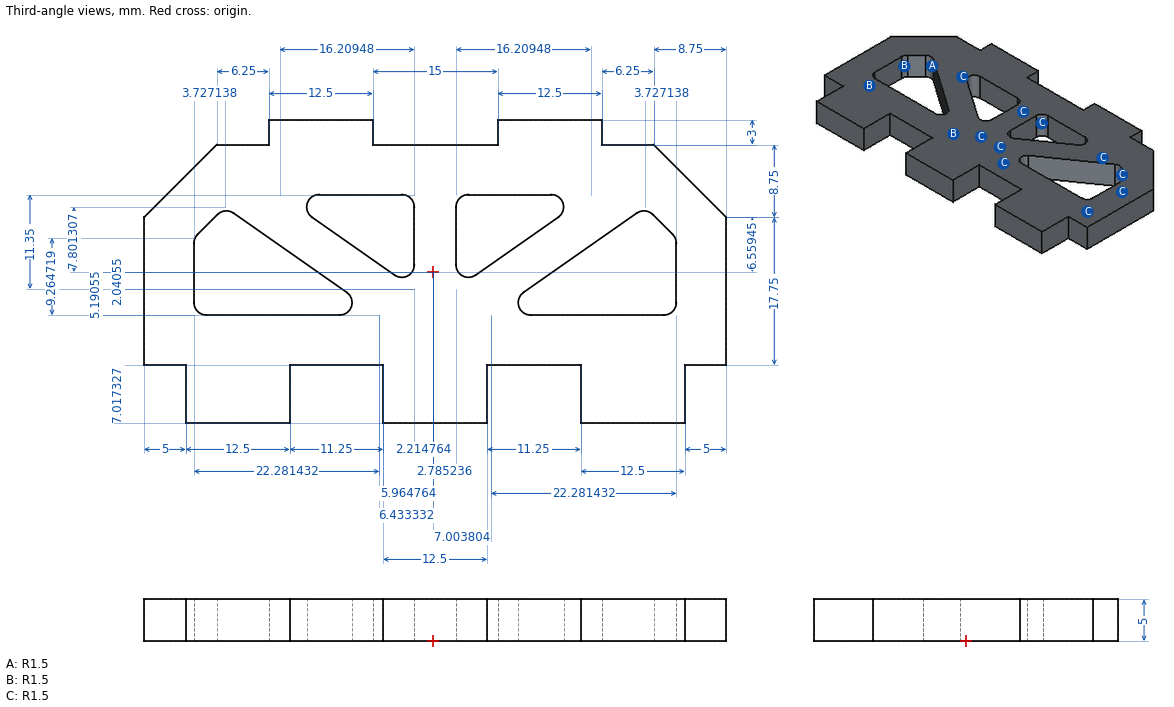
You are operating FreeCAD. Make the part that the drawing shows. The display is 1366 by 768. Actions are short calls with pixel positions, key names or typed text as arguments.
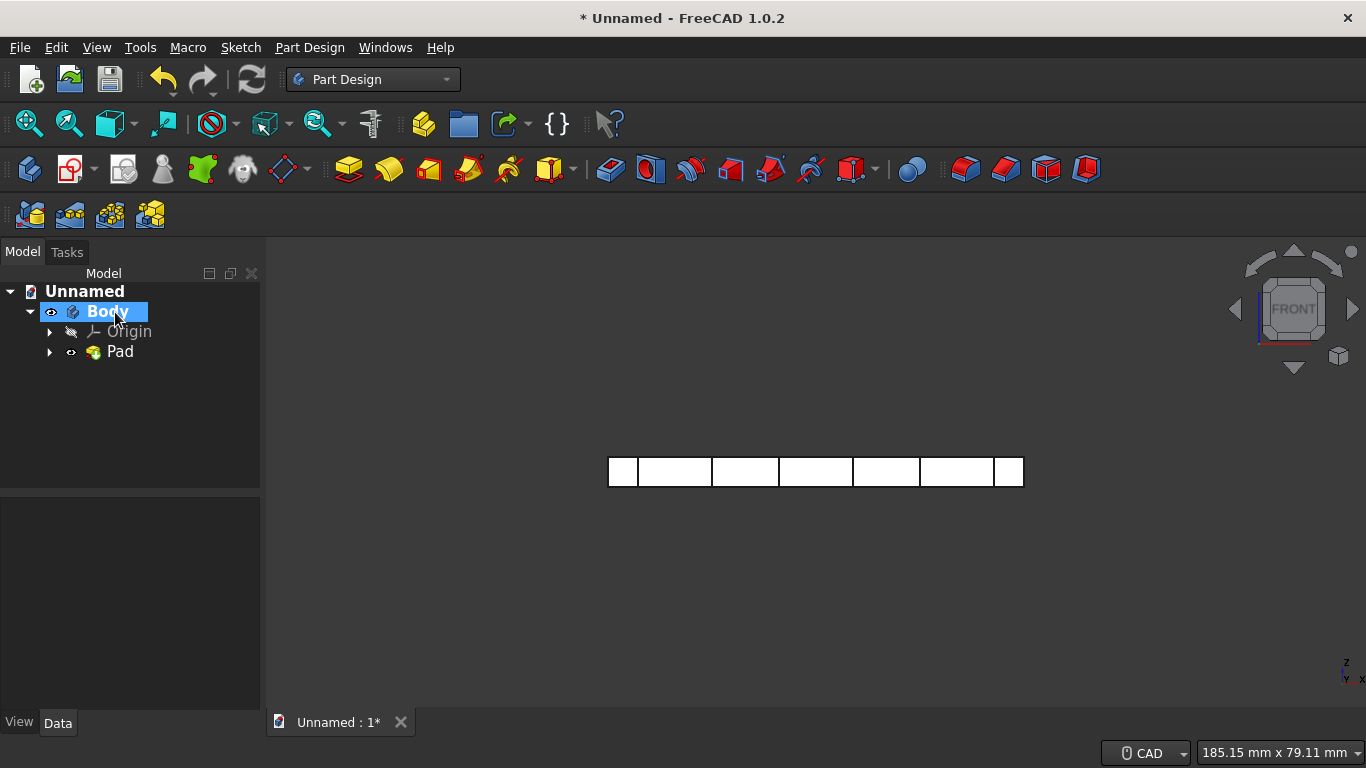
key(3)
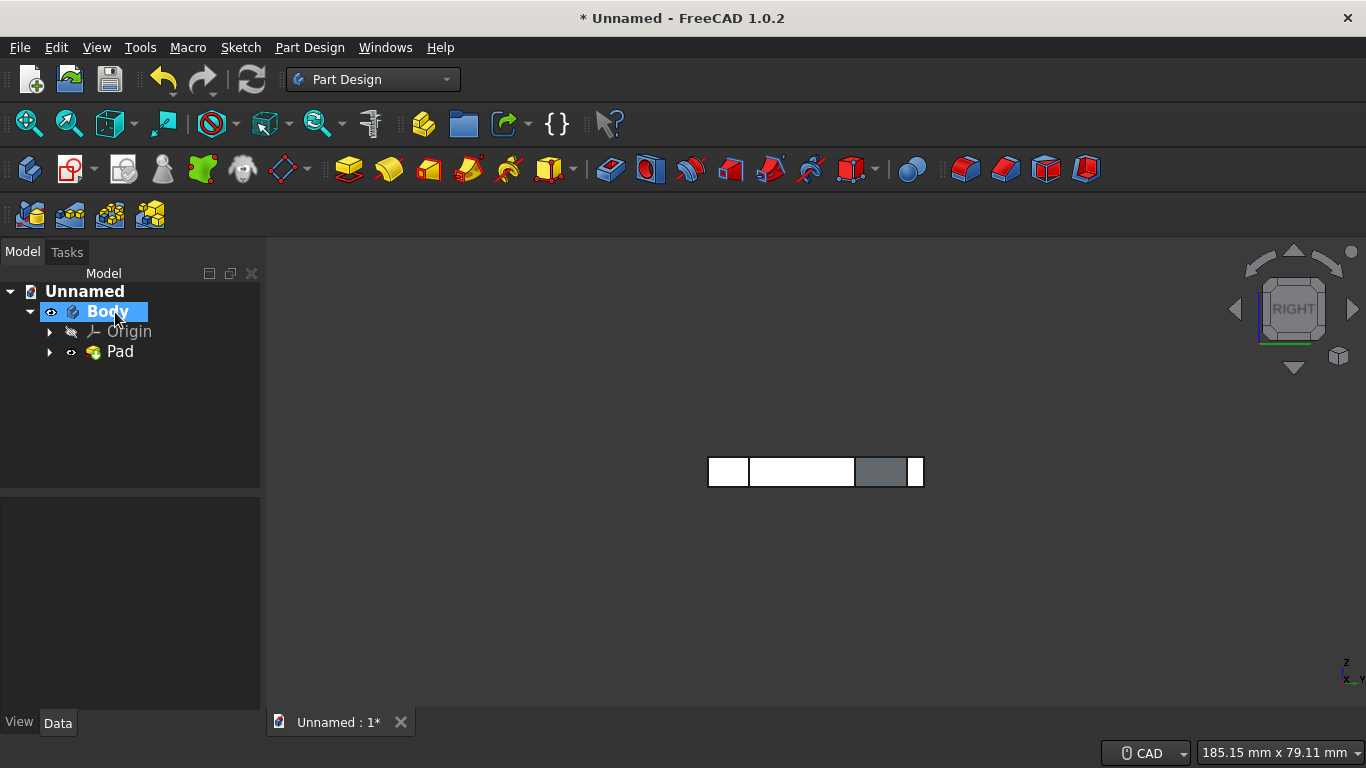
key(v)
key(f)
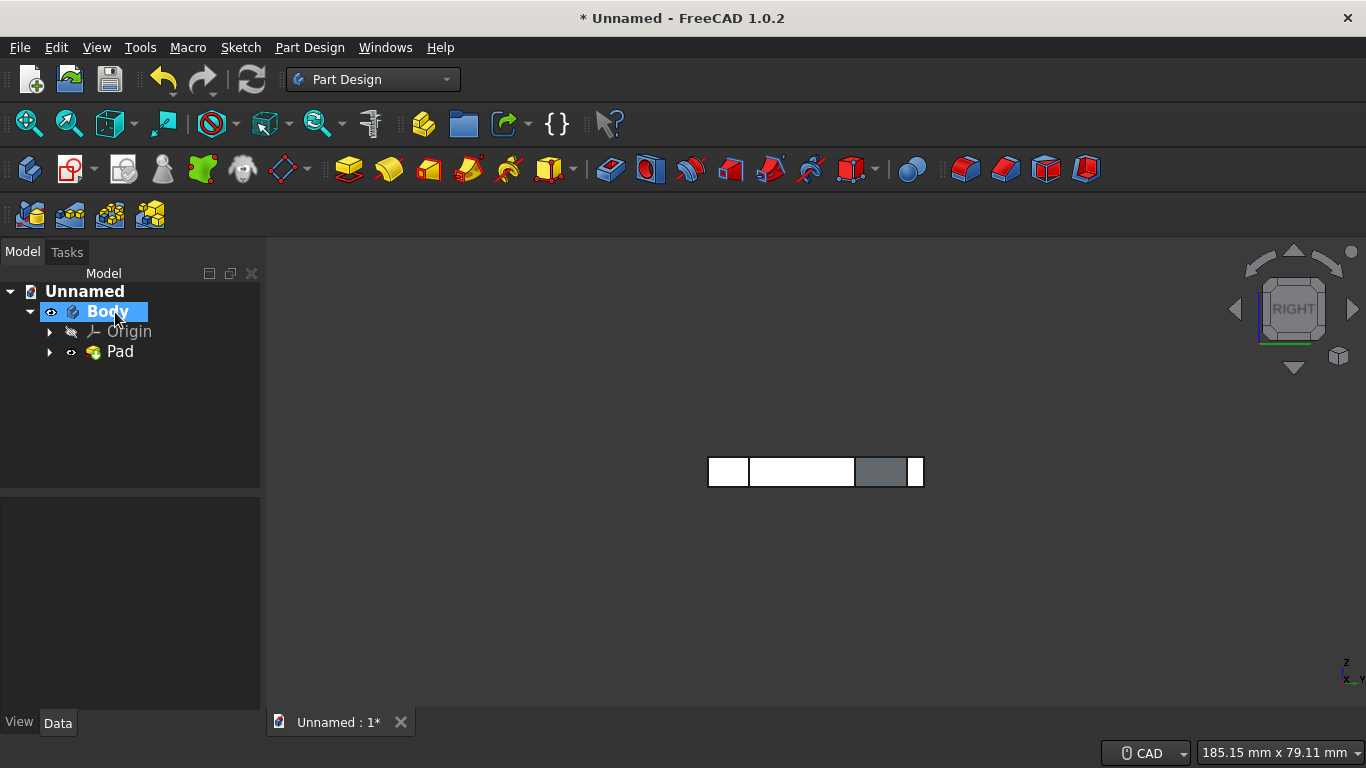
key(5)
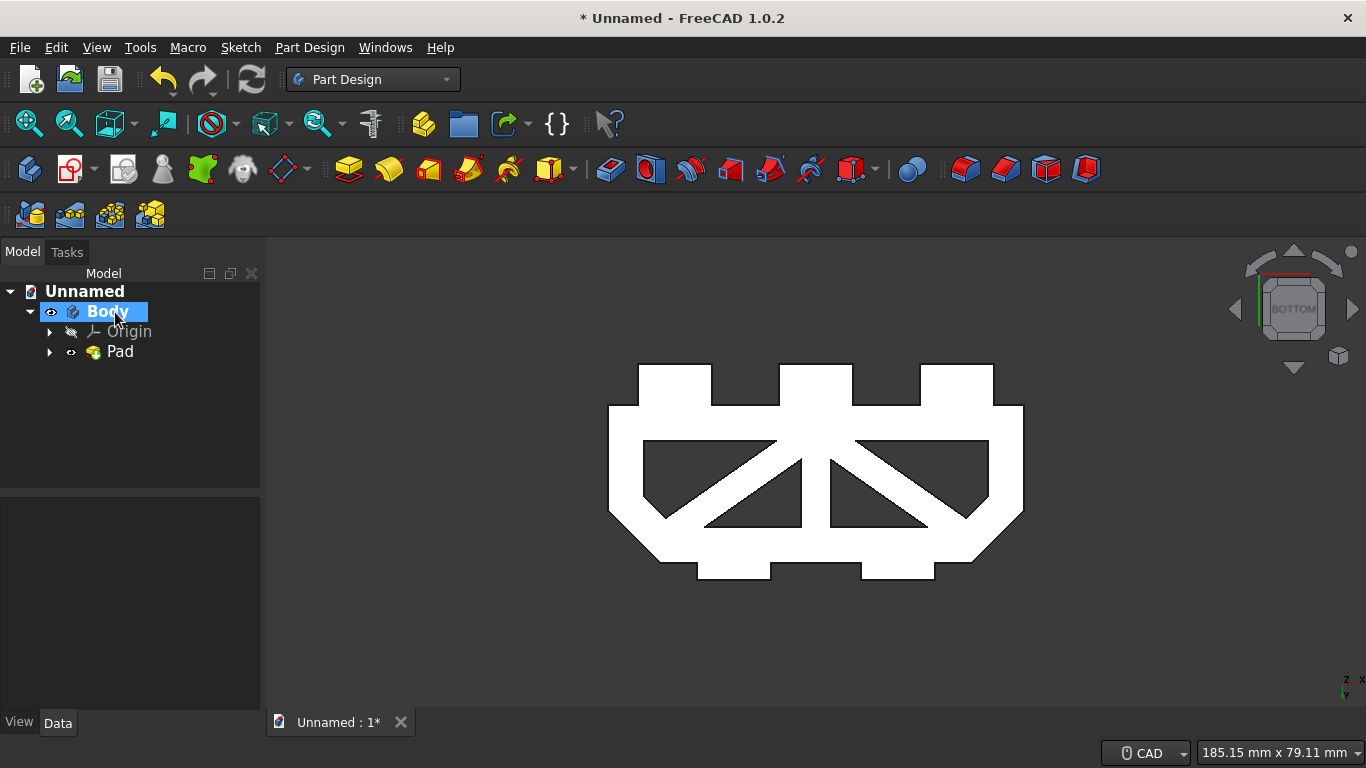
key(4)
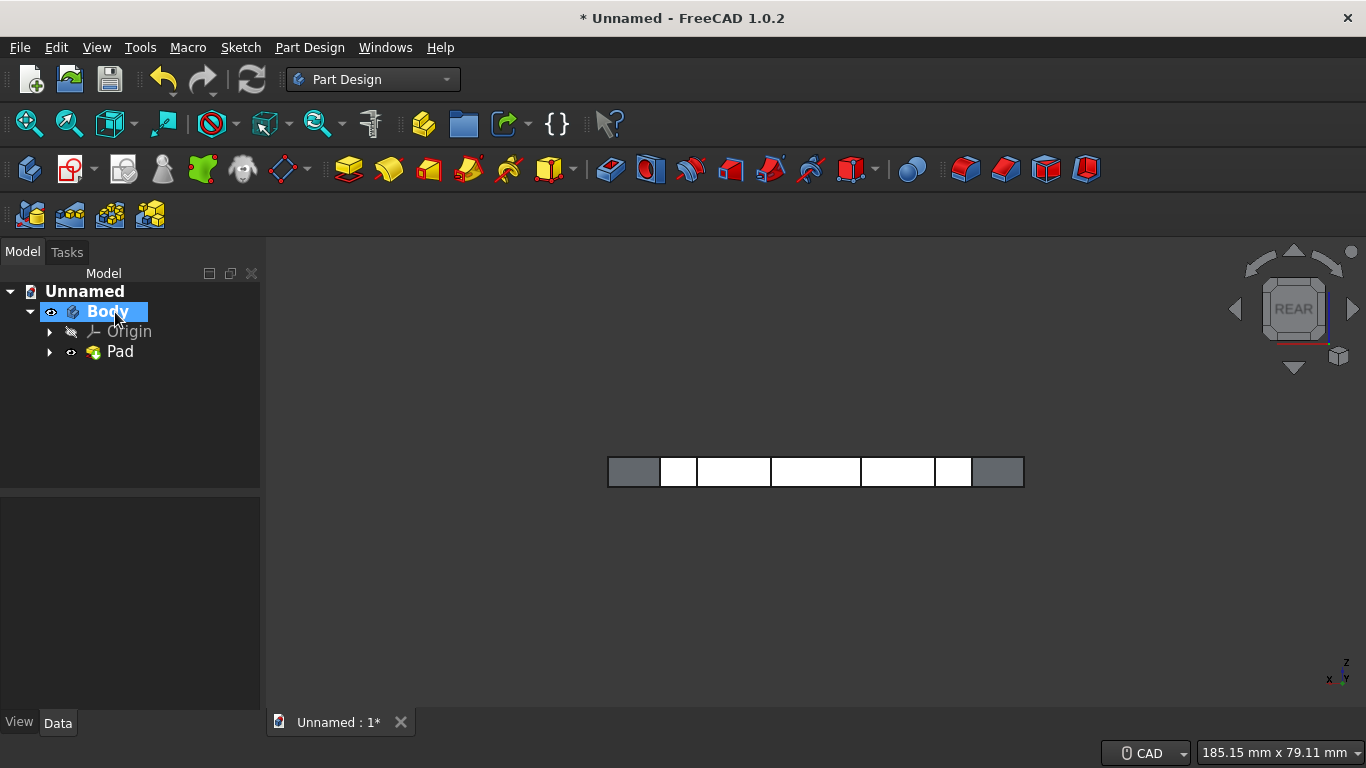
click(30, 124)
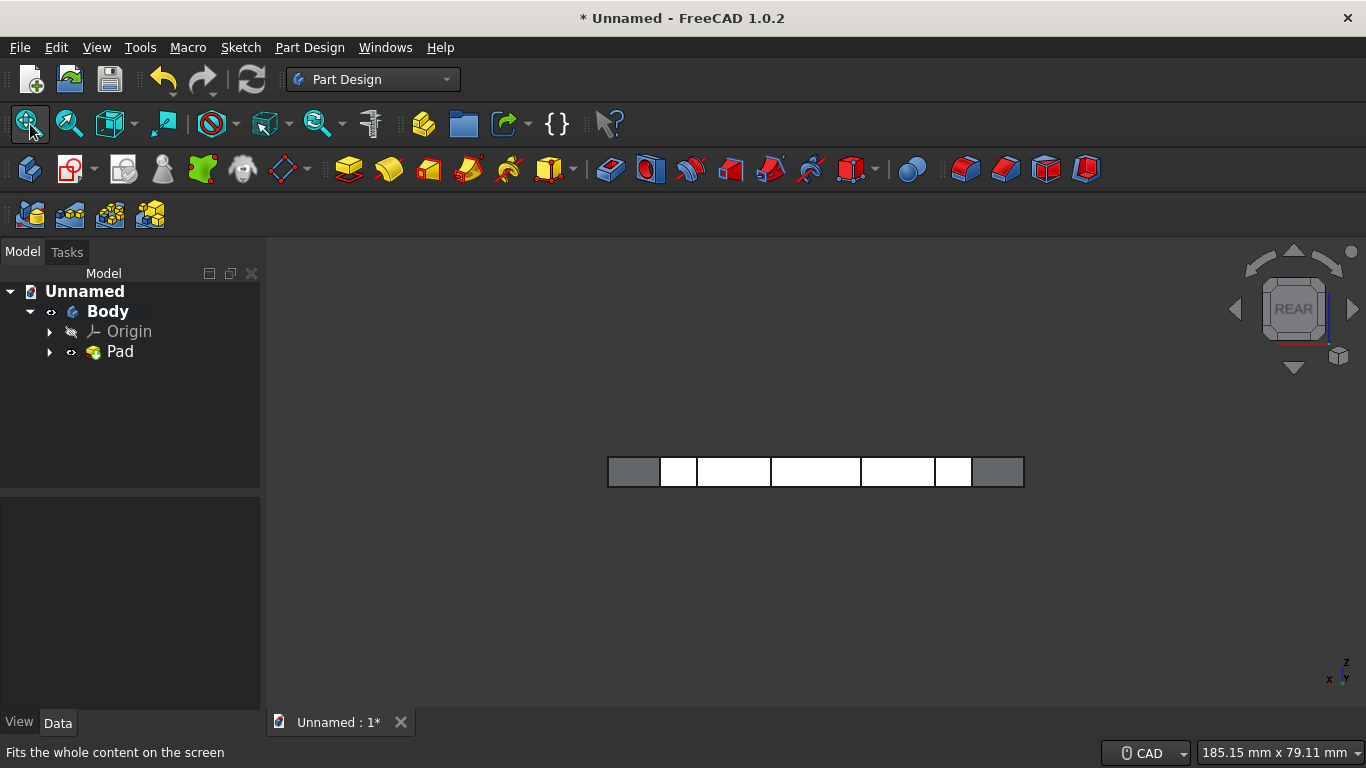
key(6)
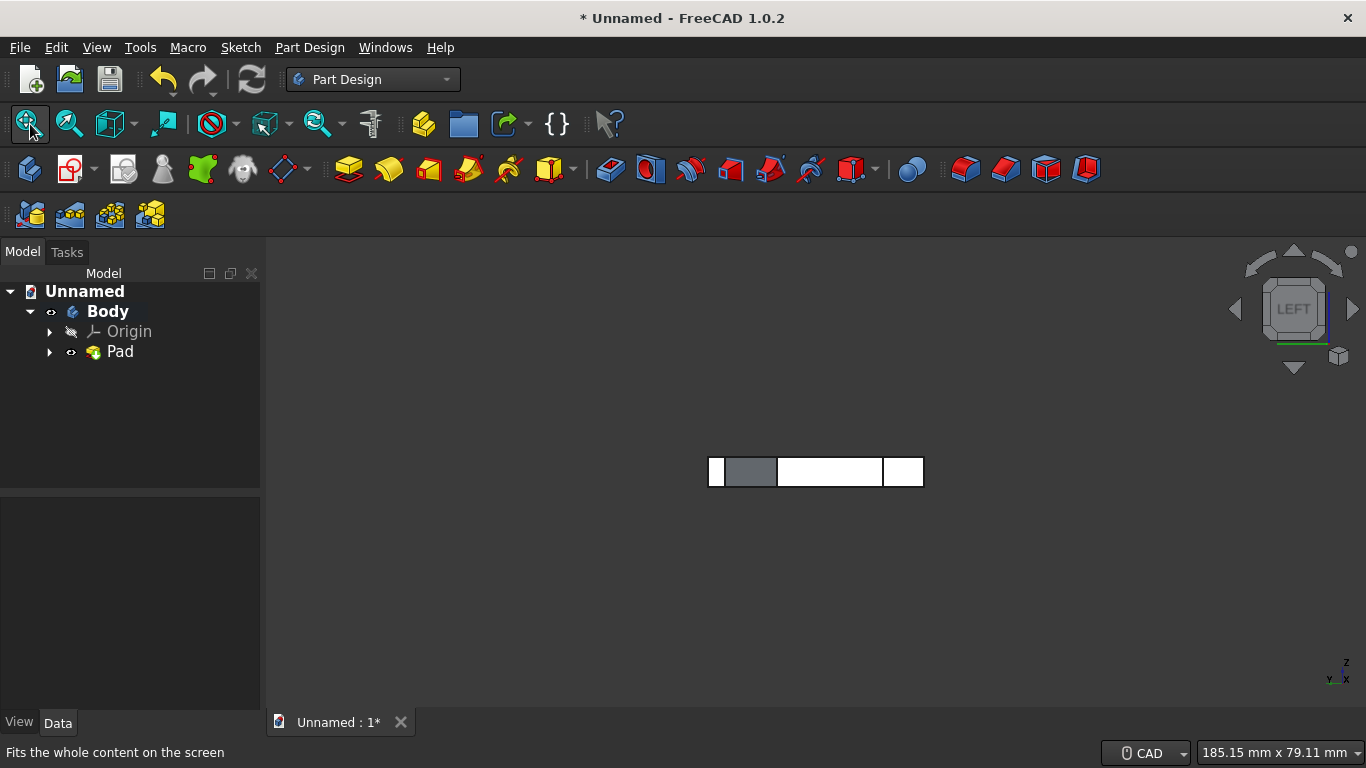
key(v)
key(f)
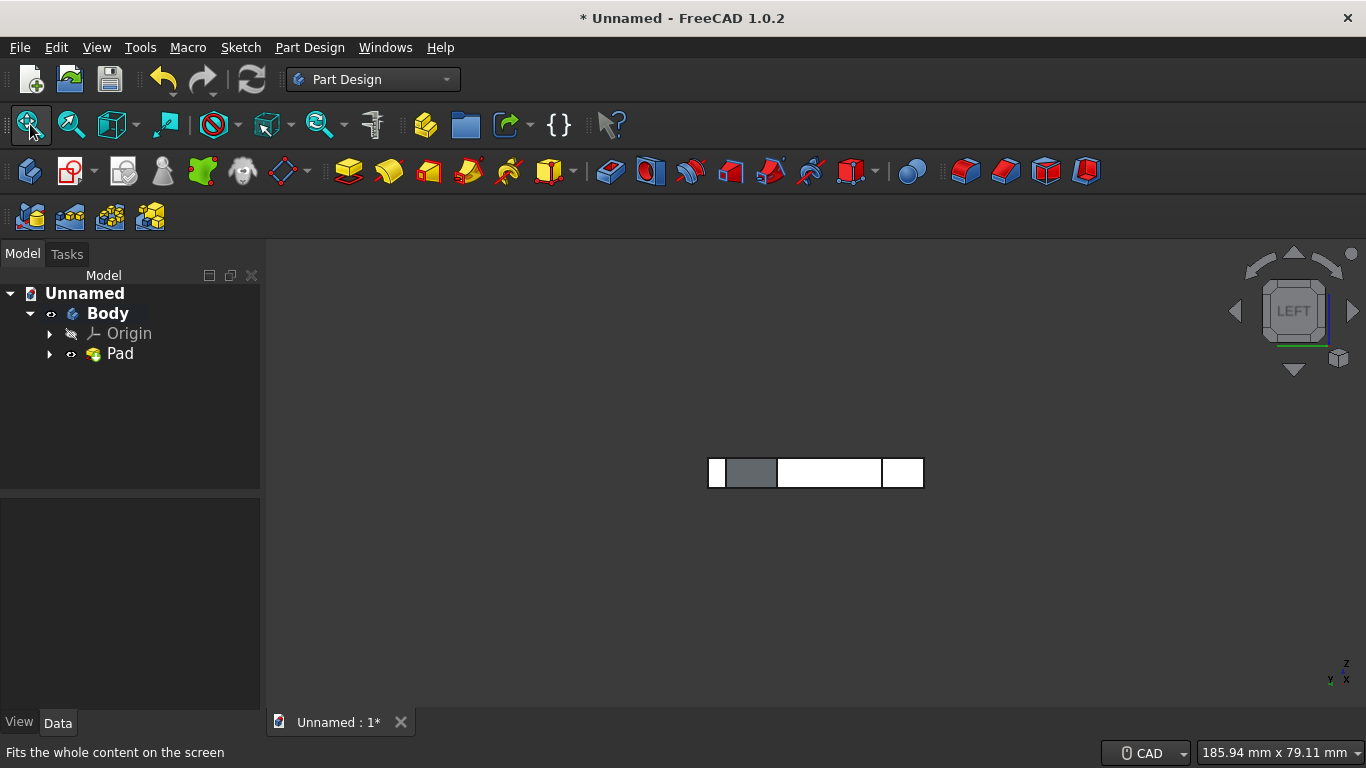
key(v)
key(3)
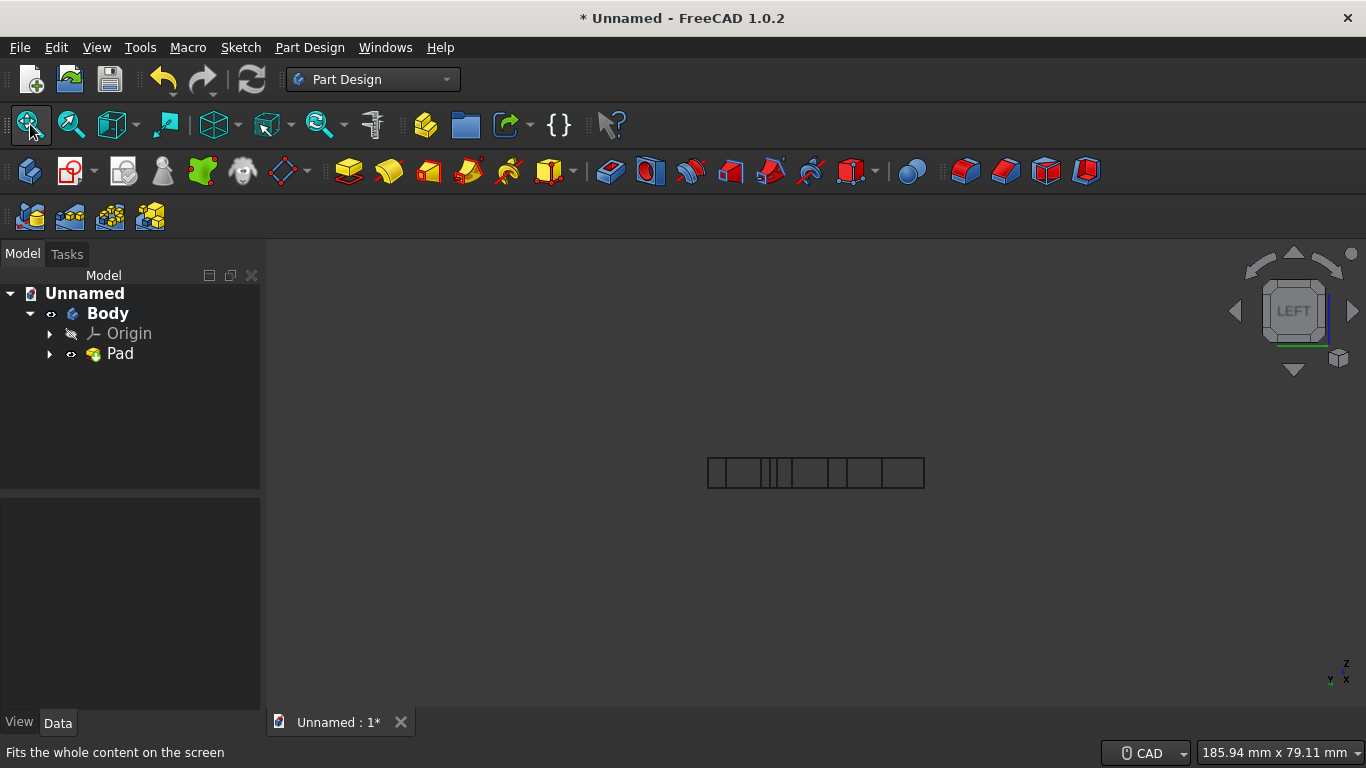
key(0)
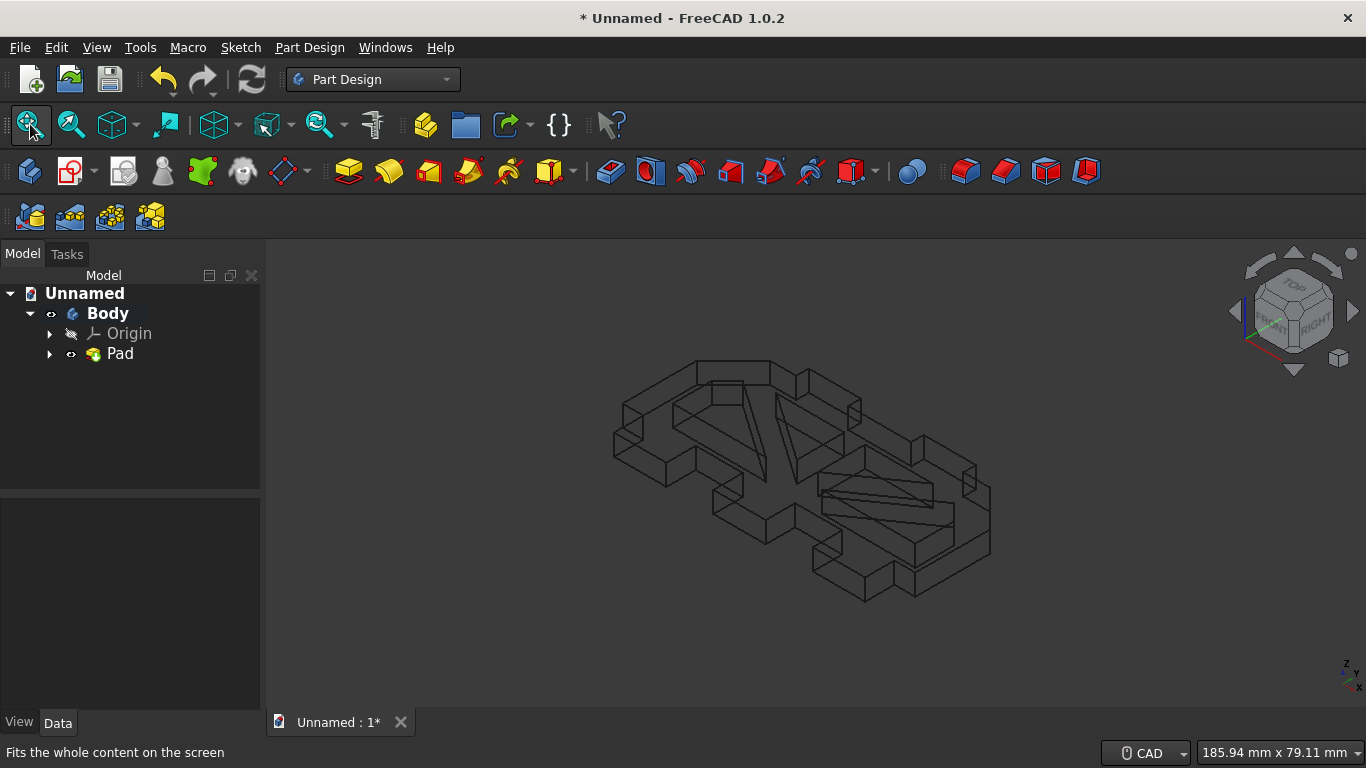
scroll(743, 392, up, 6)